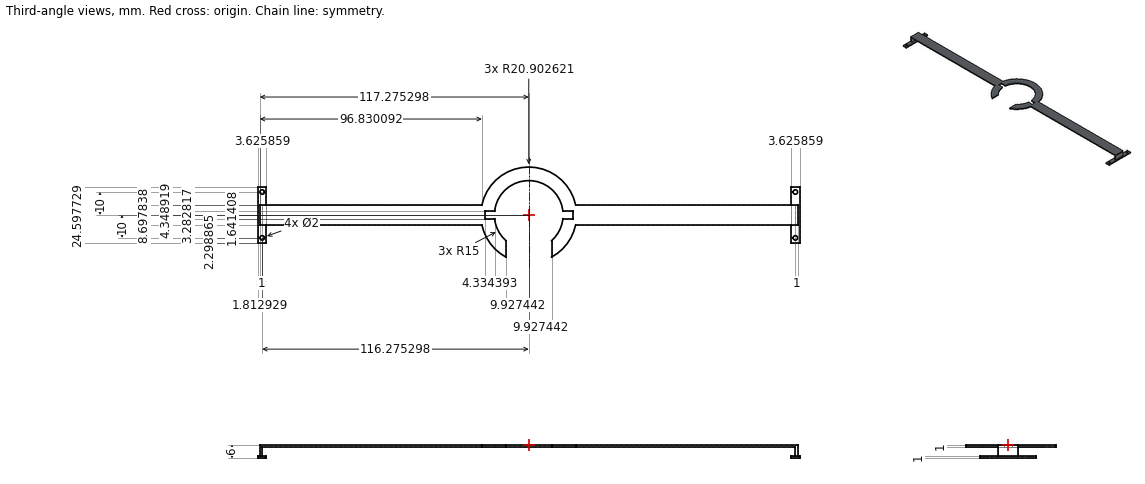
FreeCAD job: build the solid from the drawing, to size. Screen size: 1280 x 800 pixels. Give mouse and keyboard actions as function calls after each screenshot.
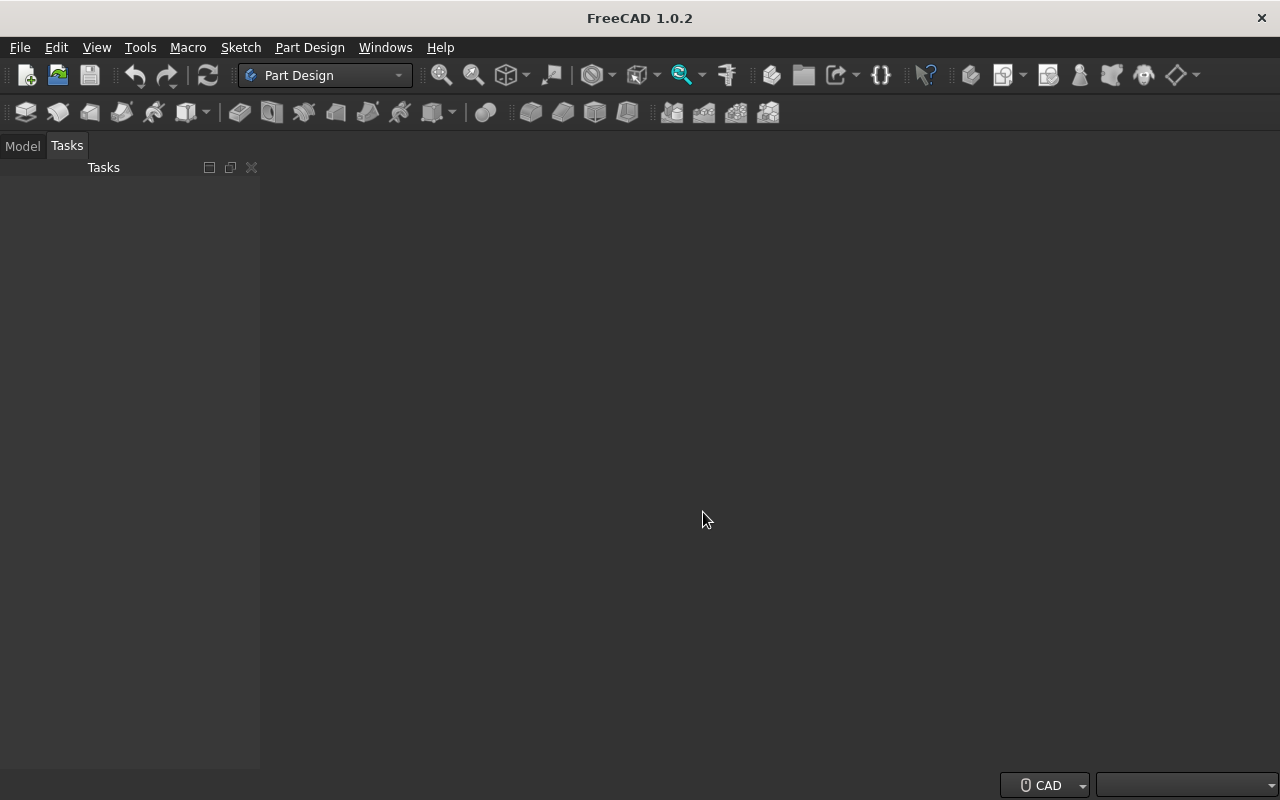
click(26, 76)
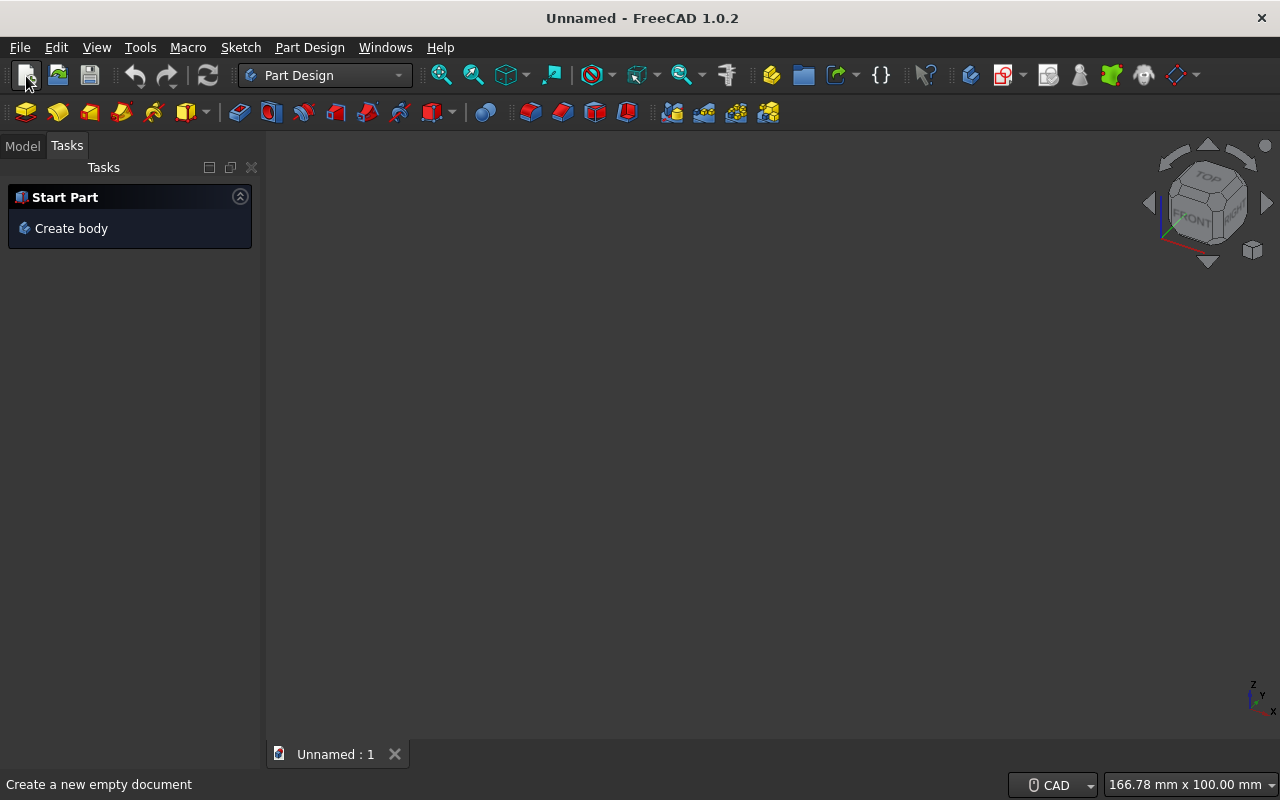
click(1004, 76)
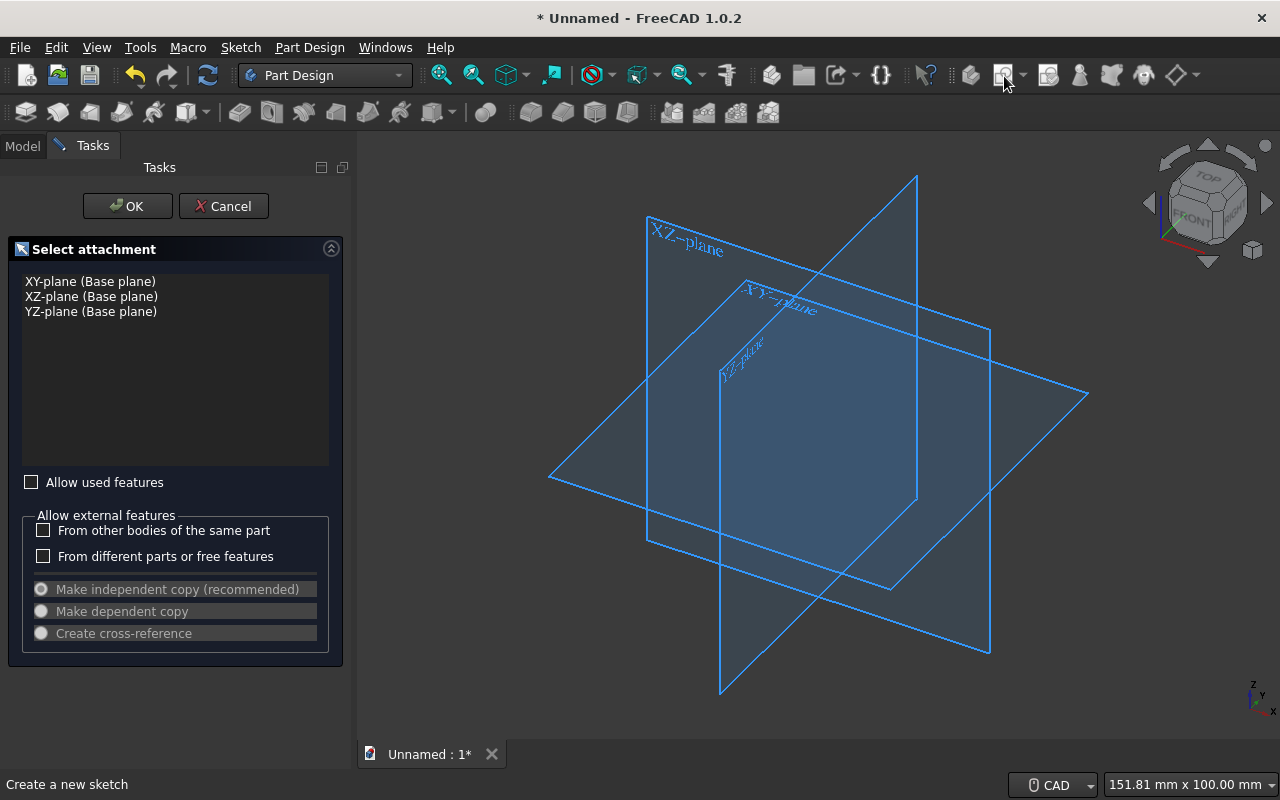
click(82, 282)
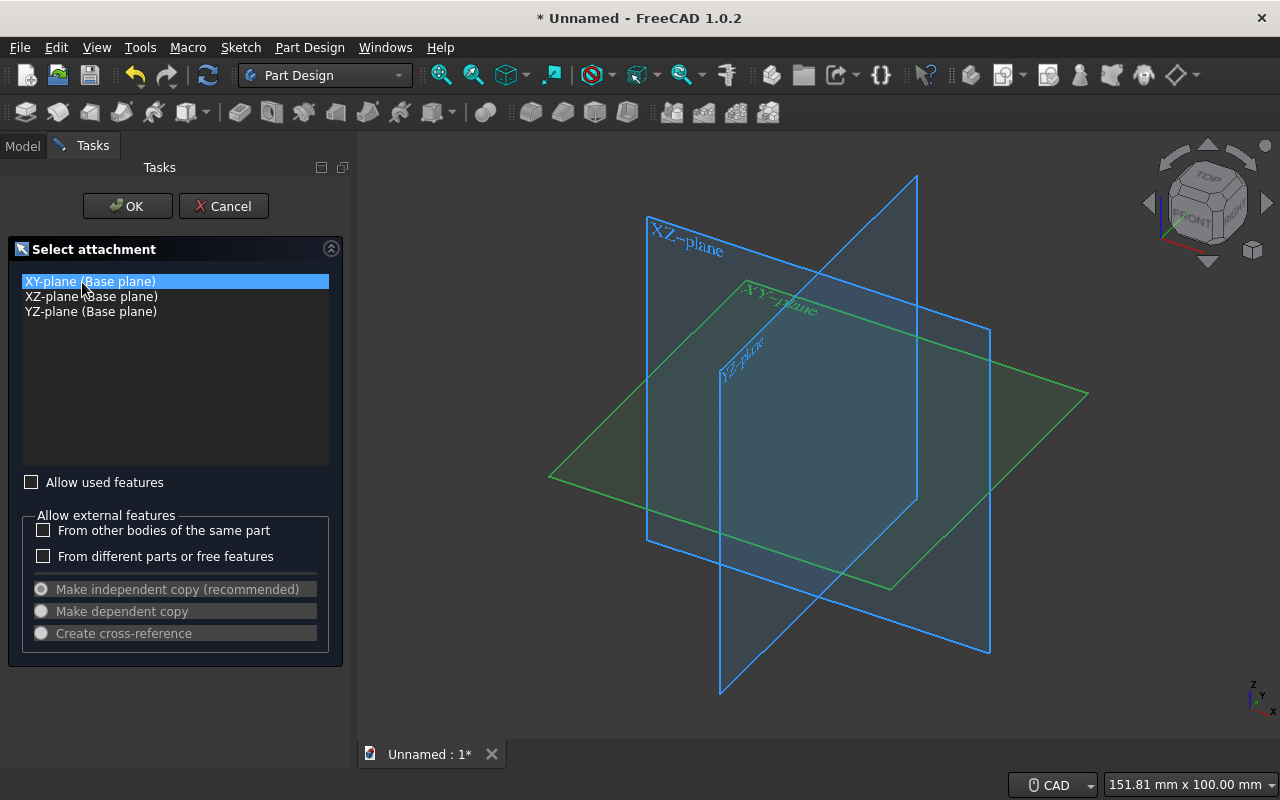
click(128, 206)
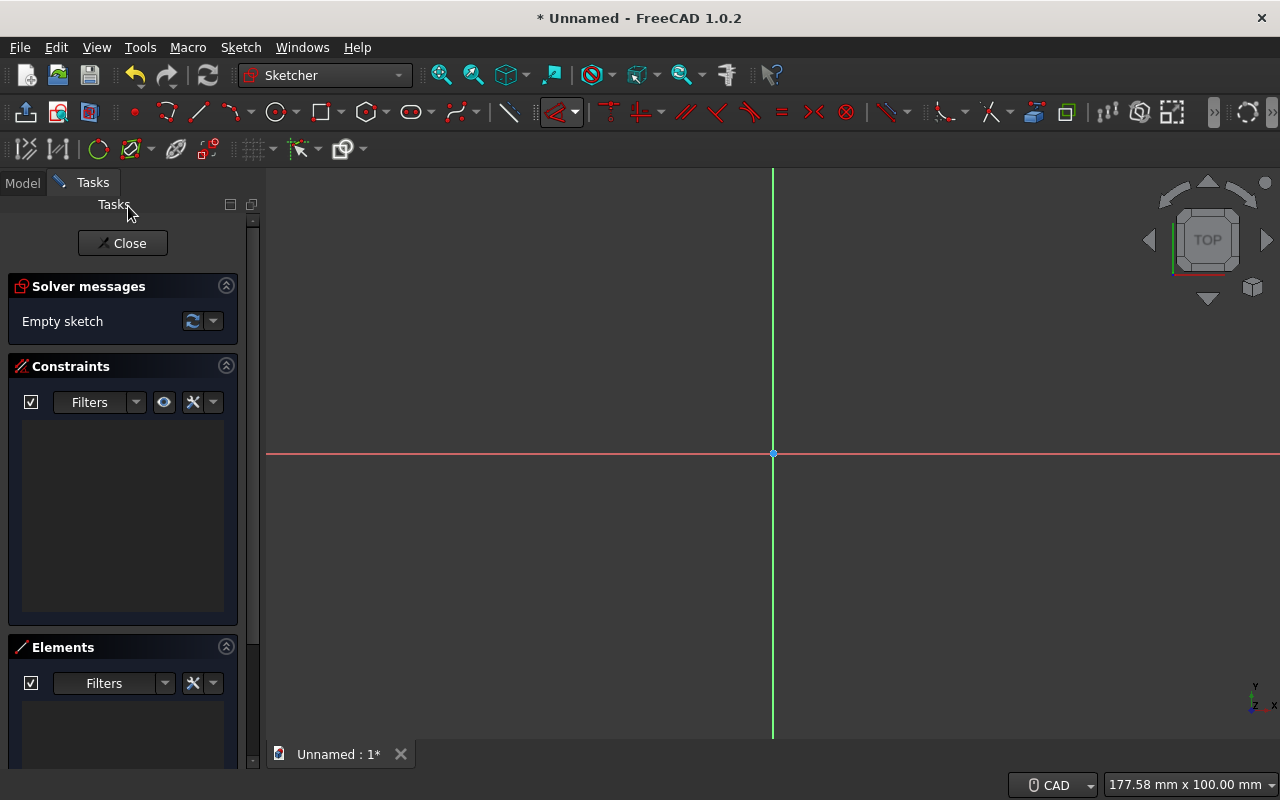
scroll(649, 459, down, 4)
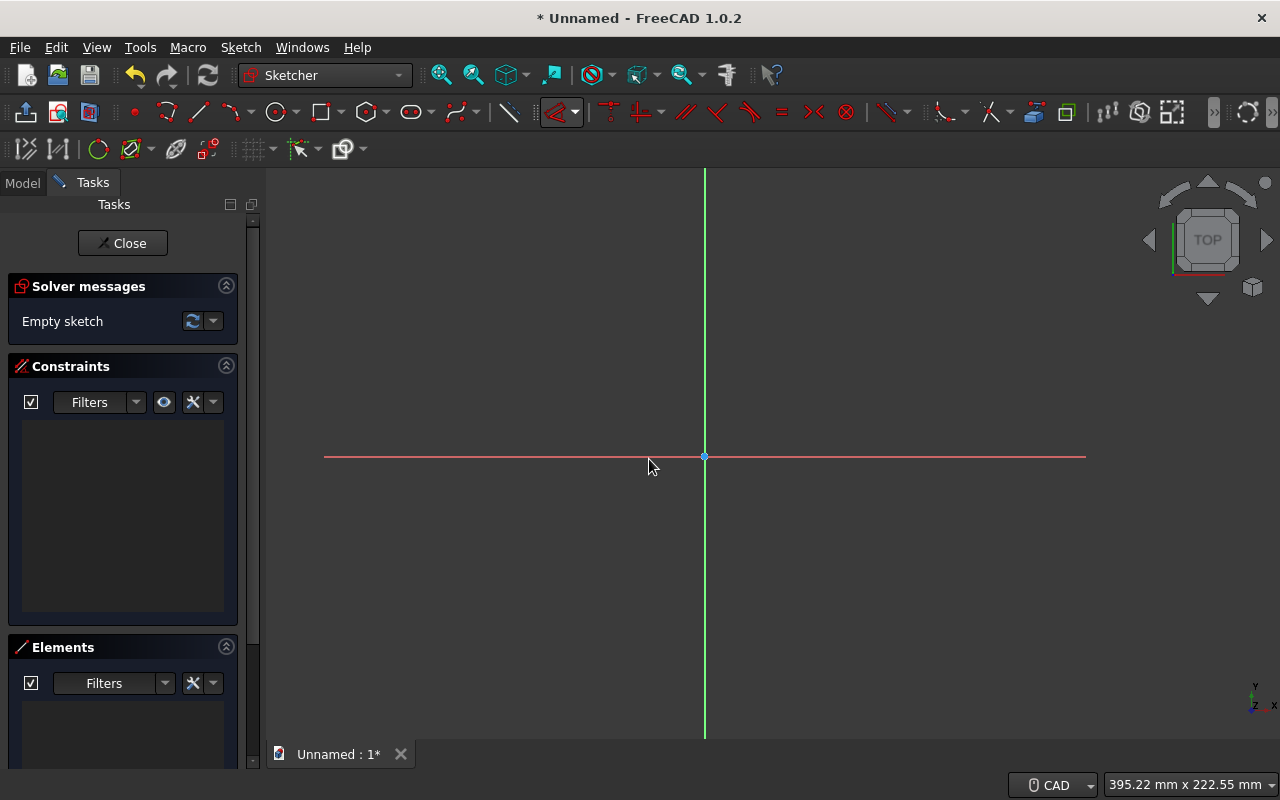
click(168, 112)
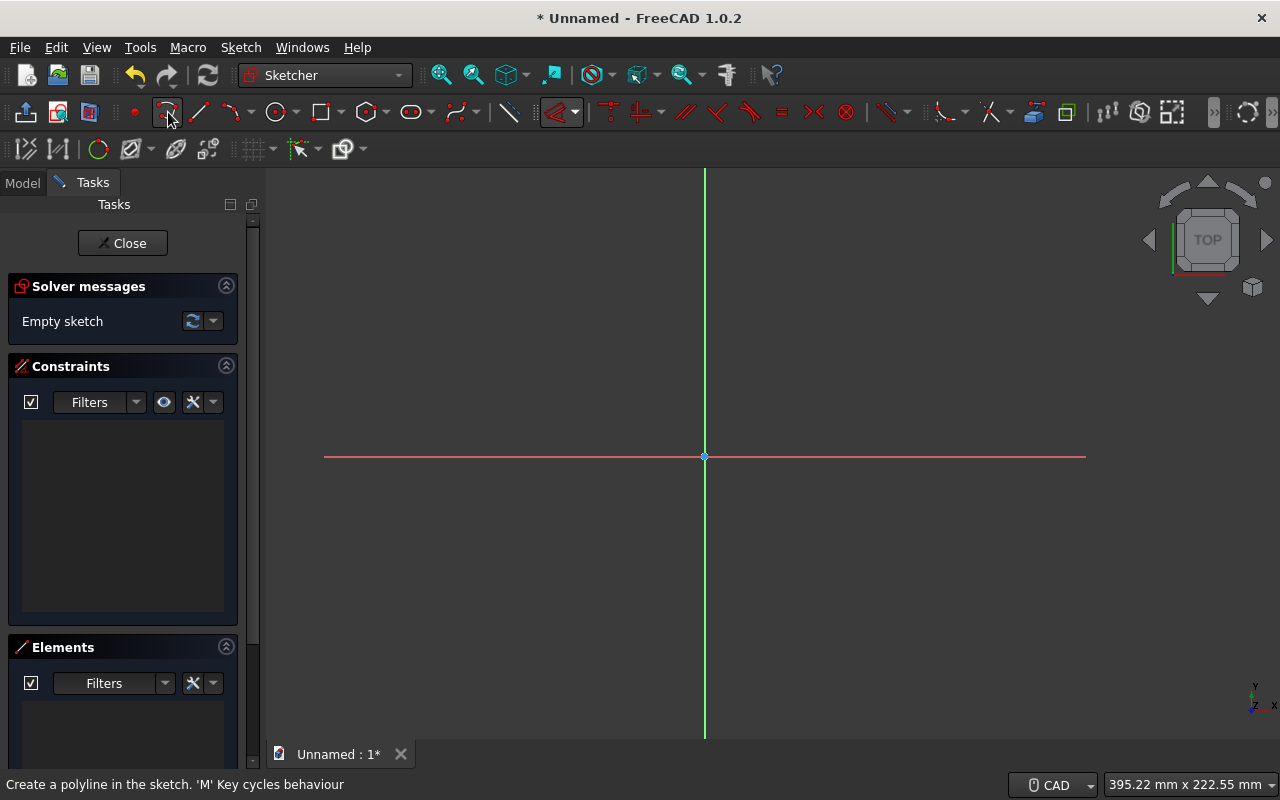
scroll(652, 446, up, 2)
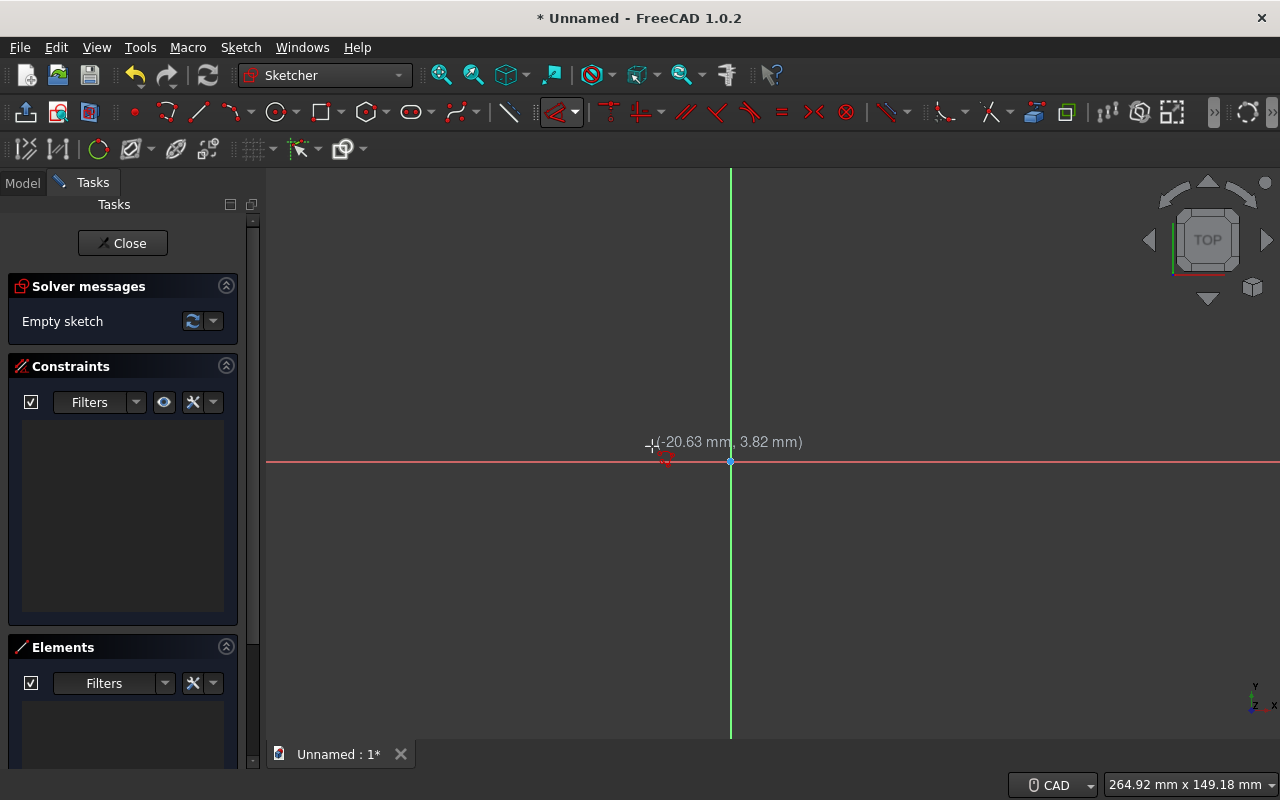
click(653, 445)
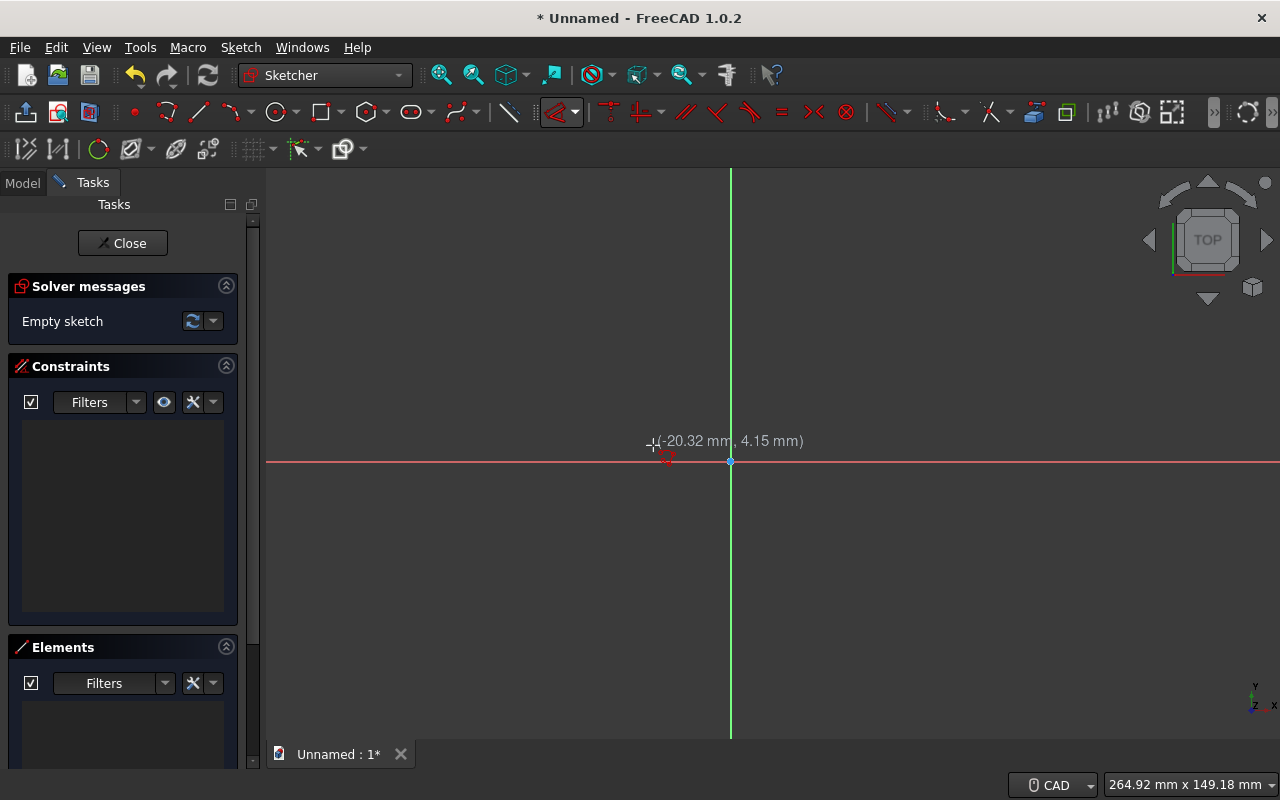
scroll(651, 446, down, 2)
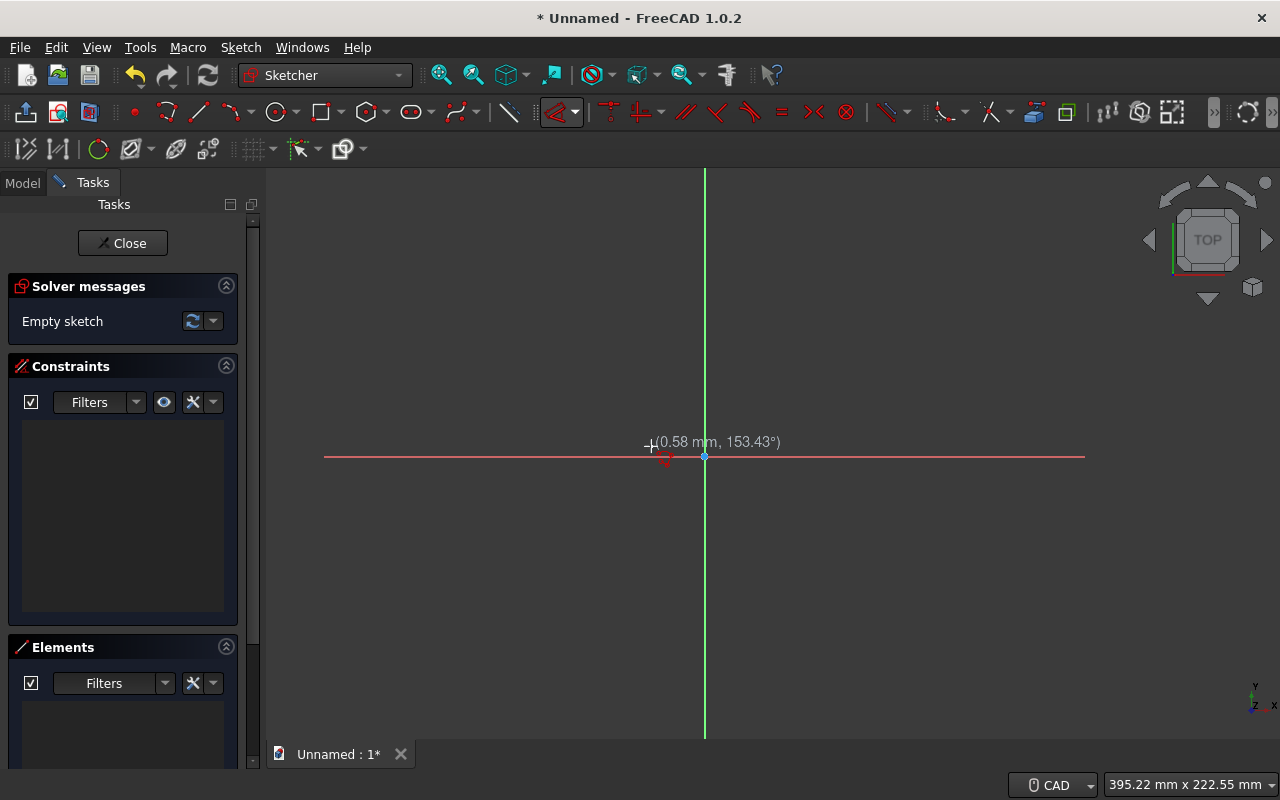
scroll(404, 446, up, 2)